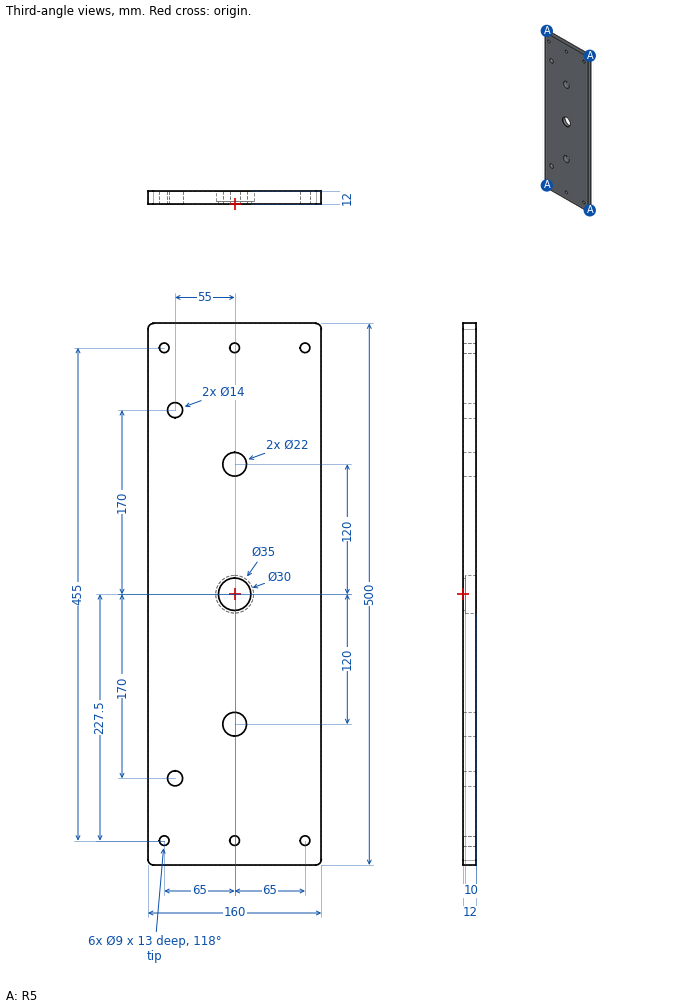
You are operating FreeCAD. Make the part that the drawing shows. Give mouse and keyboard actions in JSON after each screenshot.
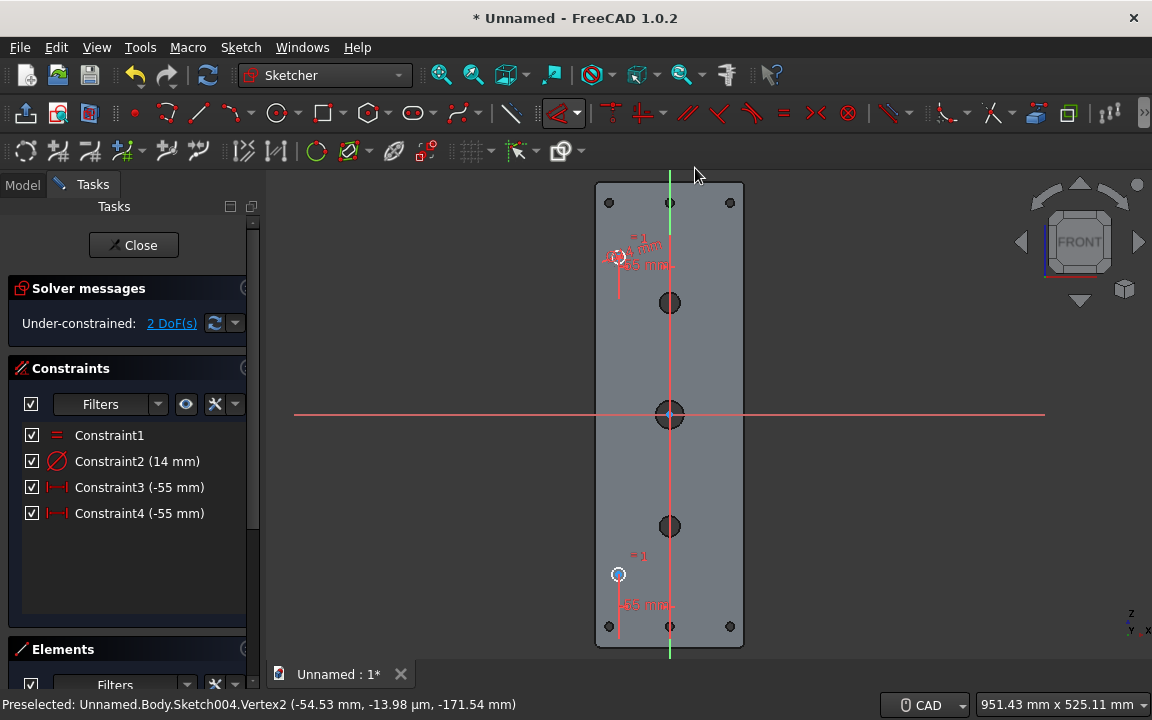
{"action": "left_click", "coordinate": [619, 257]}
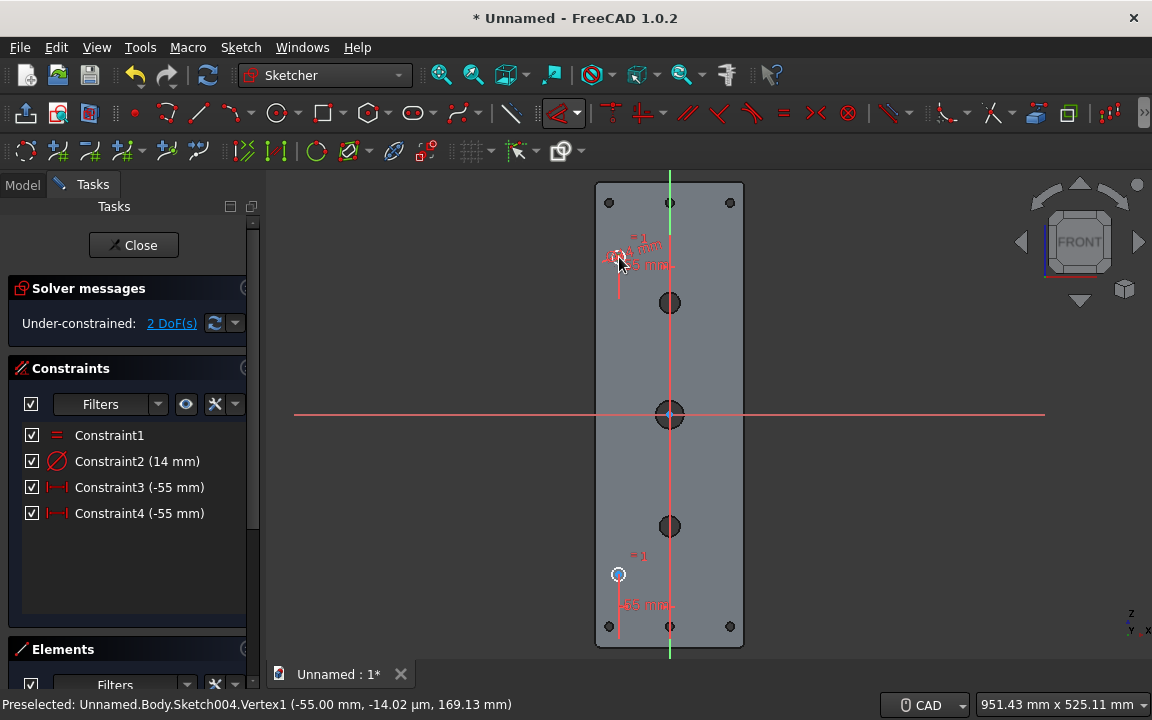
{"action": "key", "text": "i"}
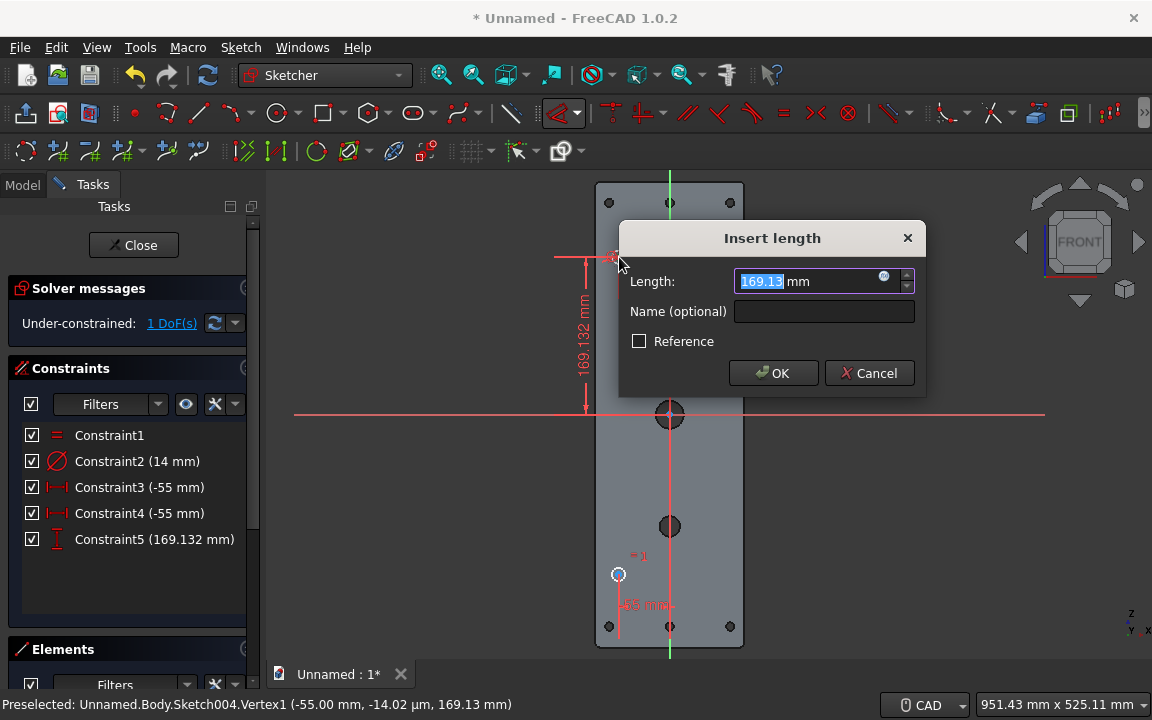
{"action": "type", "text": "170"}
{"action": "key", "text": "Return"}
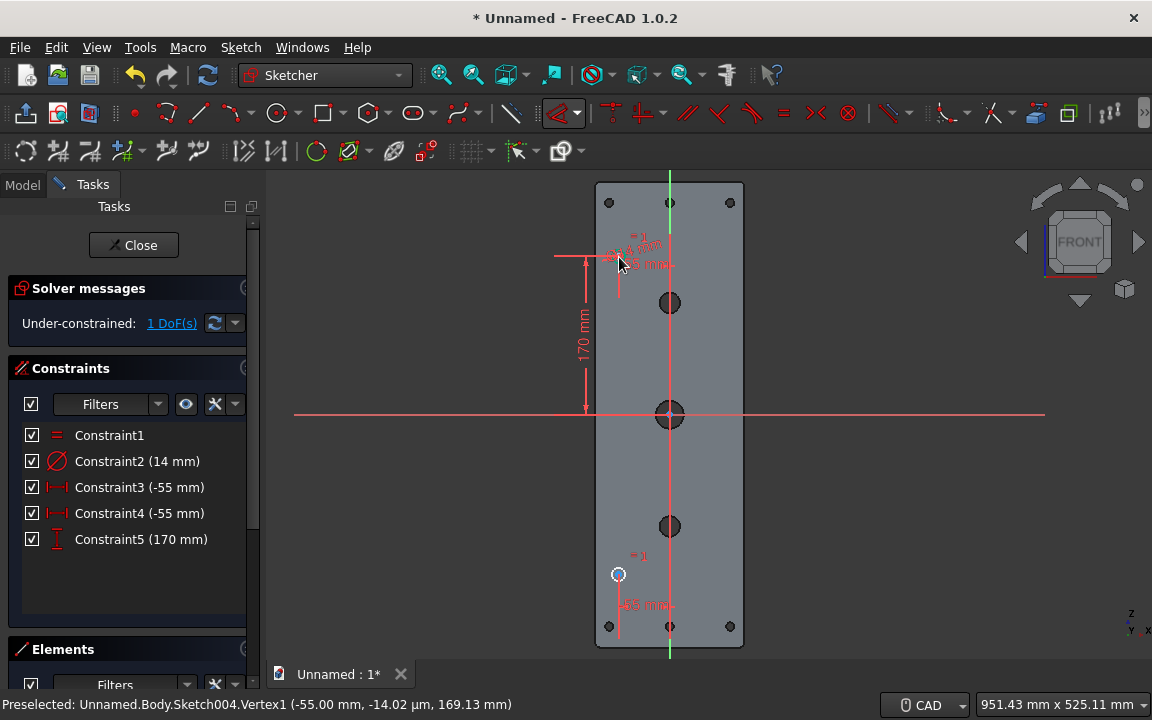
{"action": "left_click", "coordinate": [619, 574]}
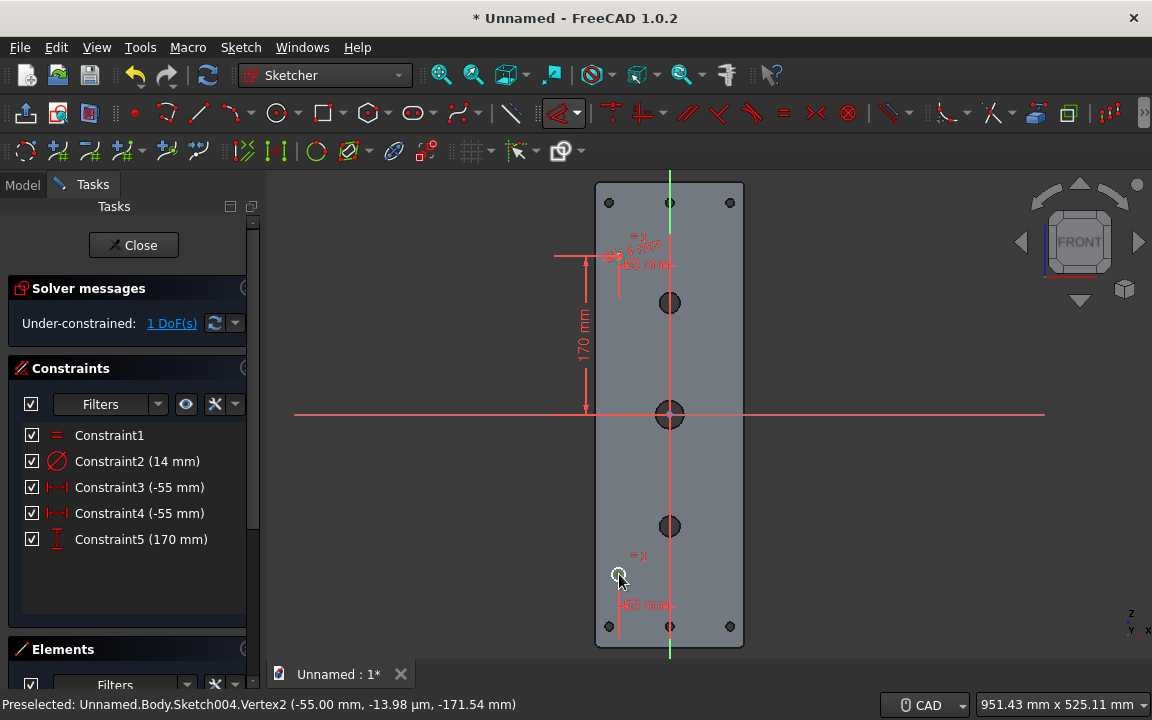
{"action": "left_click", "coordinate": [580, 114]}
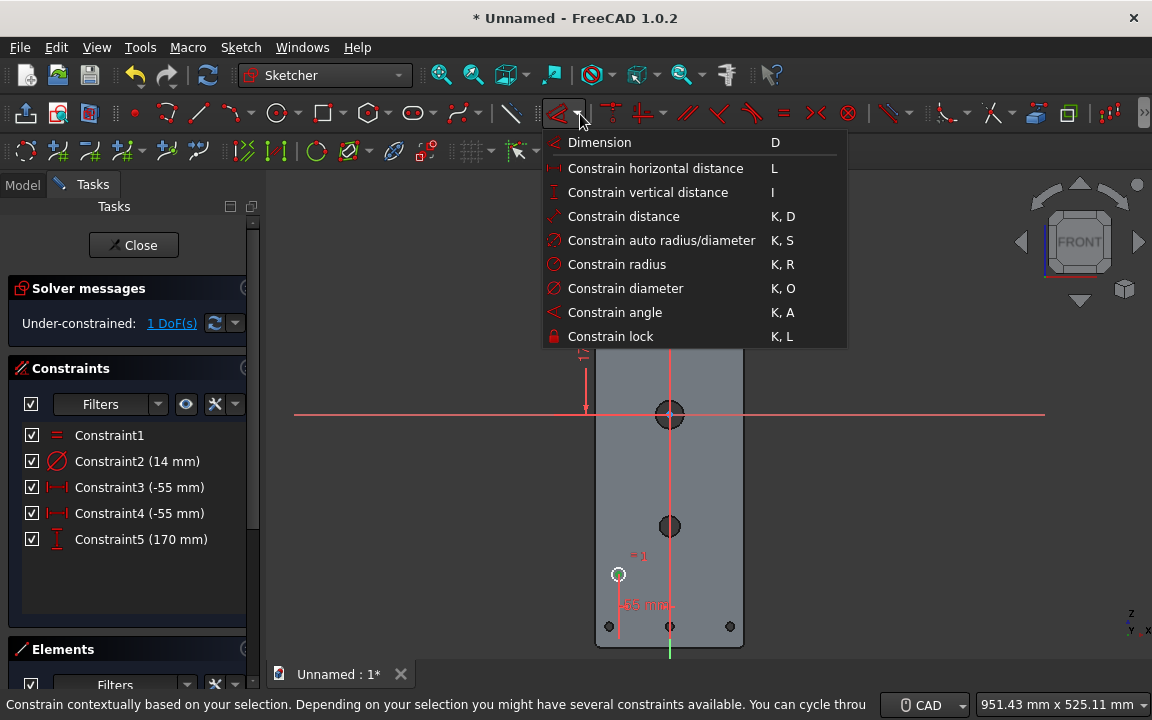
{"action": "left_click", "coordinate": [695, 192]}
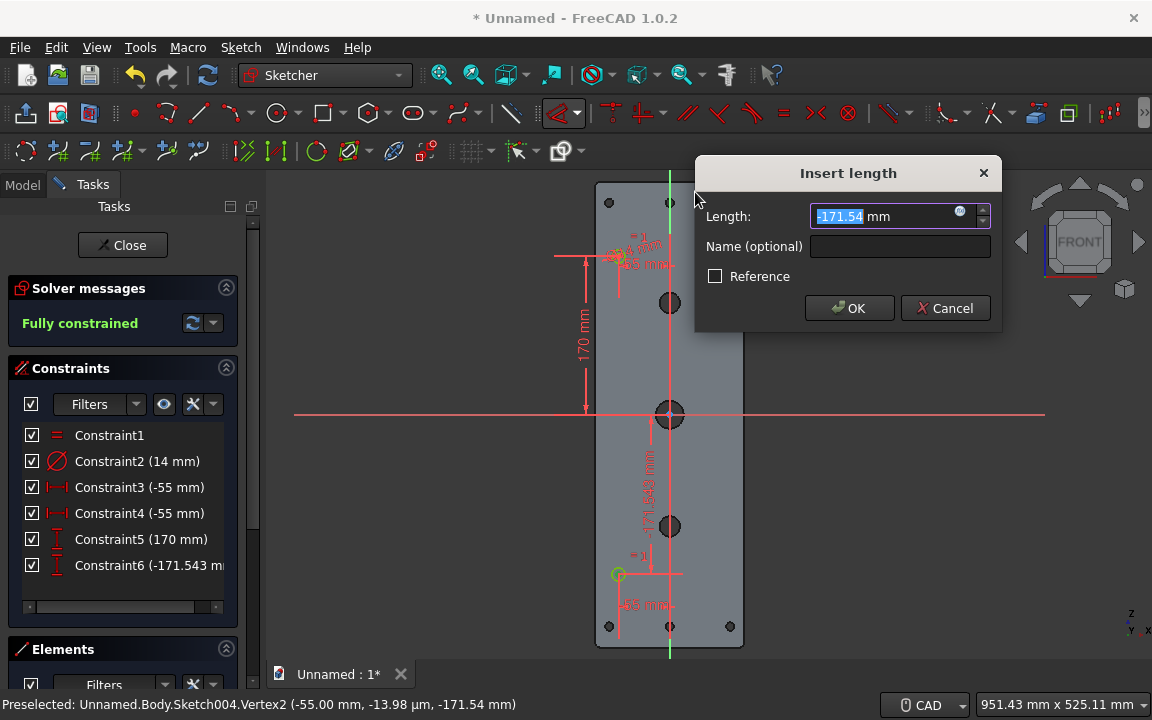
{"action": "type", "text": "-170"}
{"action": "key", "text": "Return"}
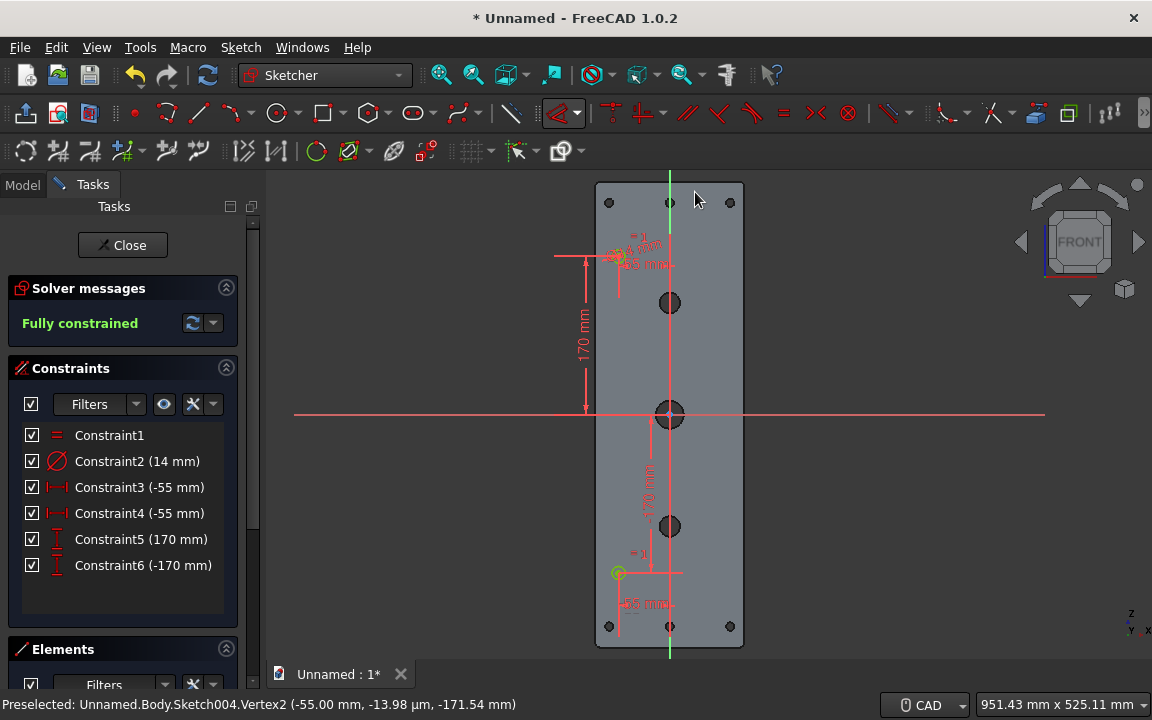
{"action": "left_click", "coordinate": [123, 245]}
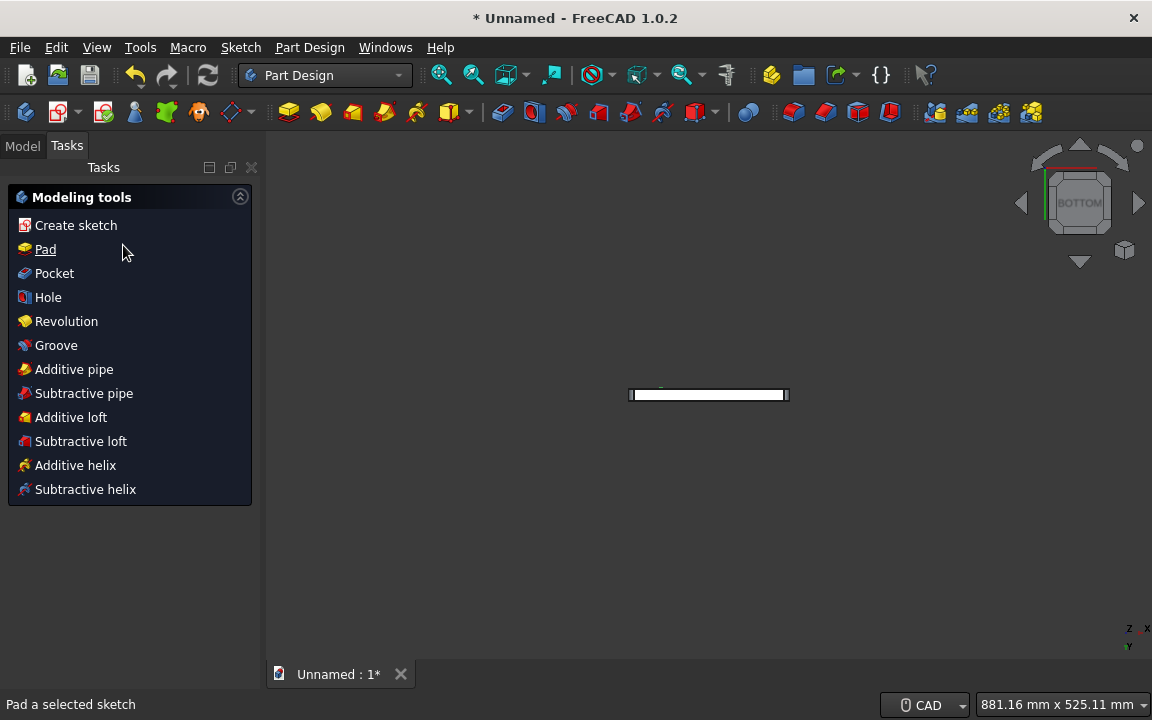
{"action": "left_click", "coordinate": [504, 112]}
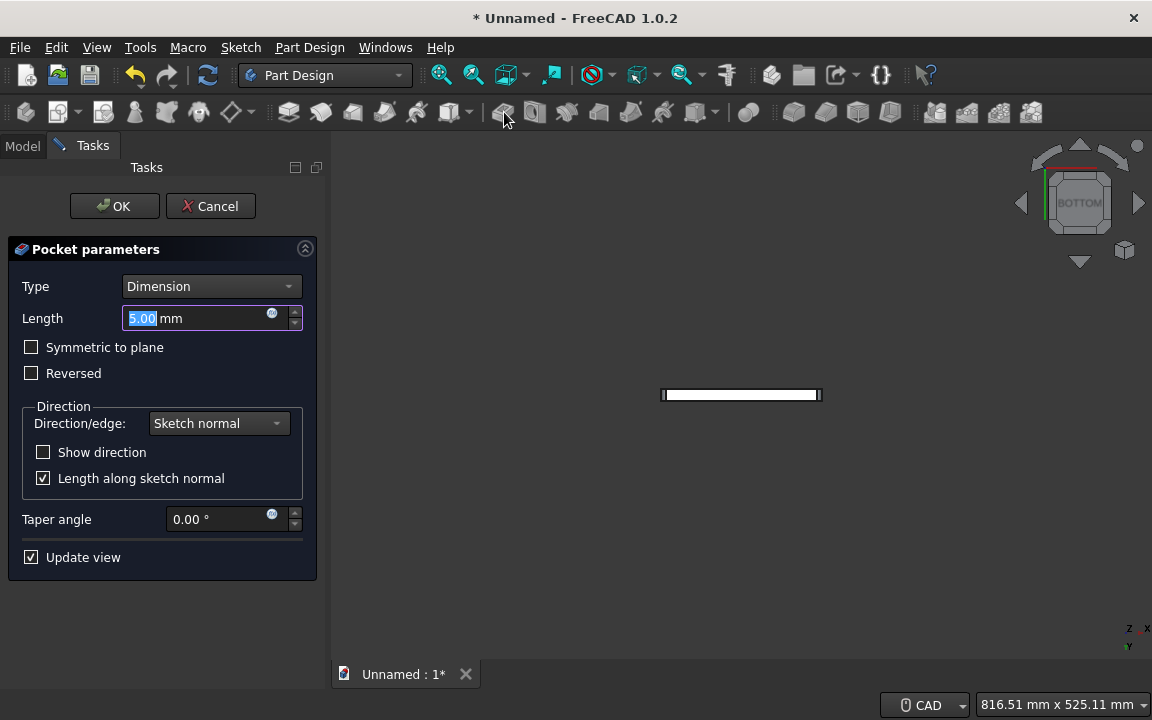
{"action": "left_click", "coordinate": [212, 286]}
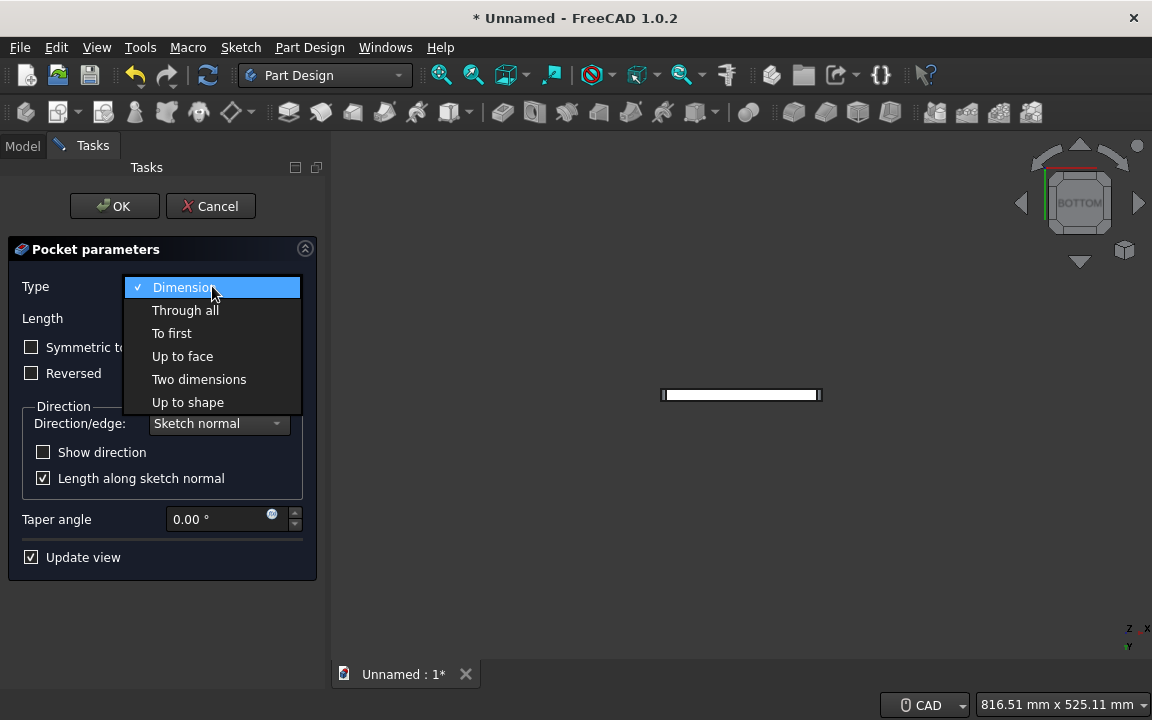
{"action": "left_click", "coordinate": [212, 310]}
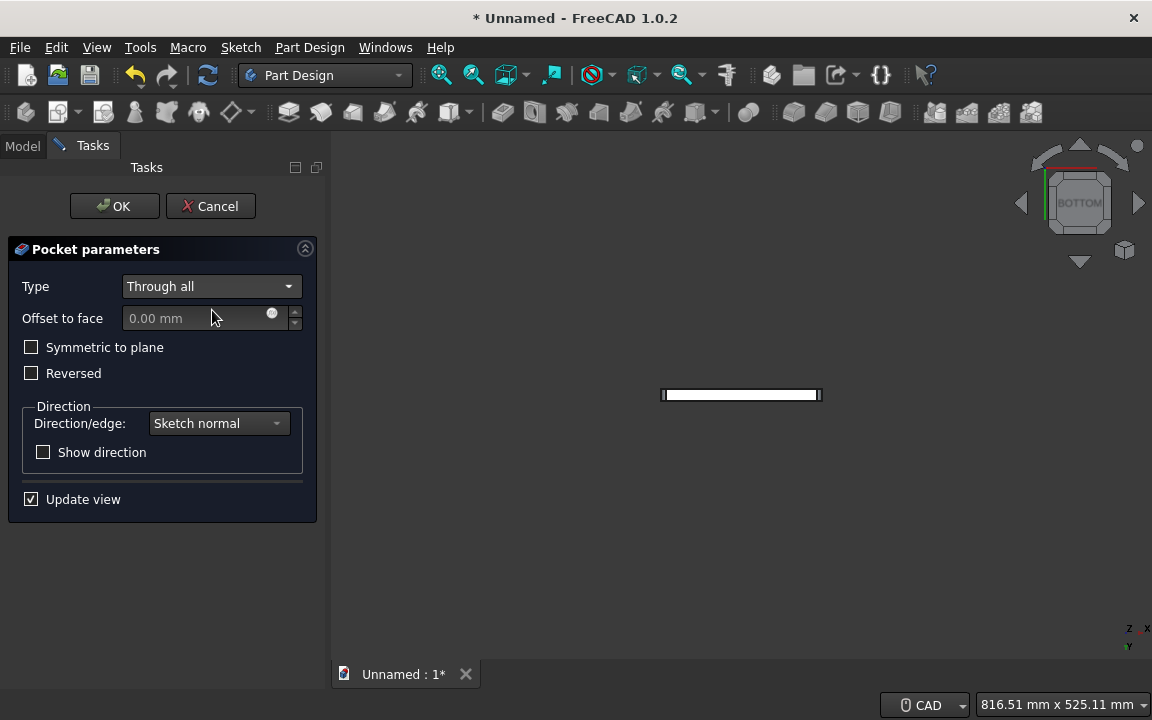
{"action": "left_click", "coordinate": [115, 206]}